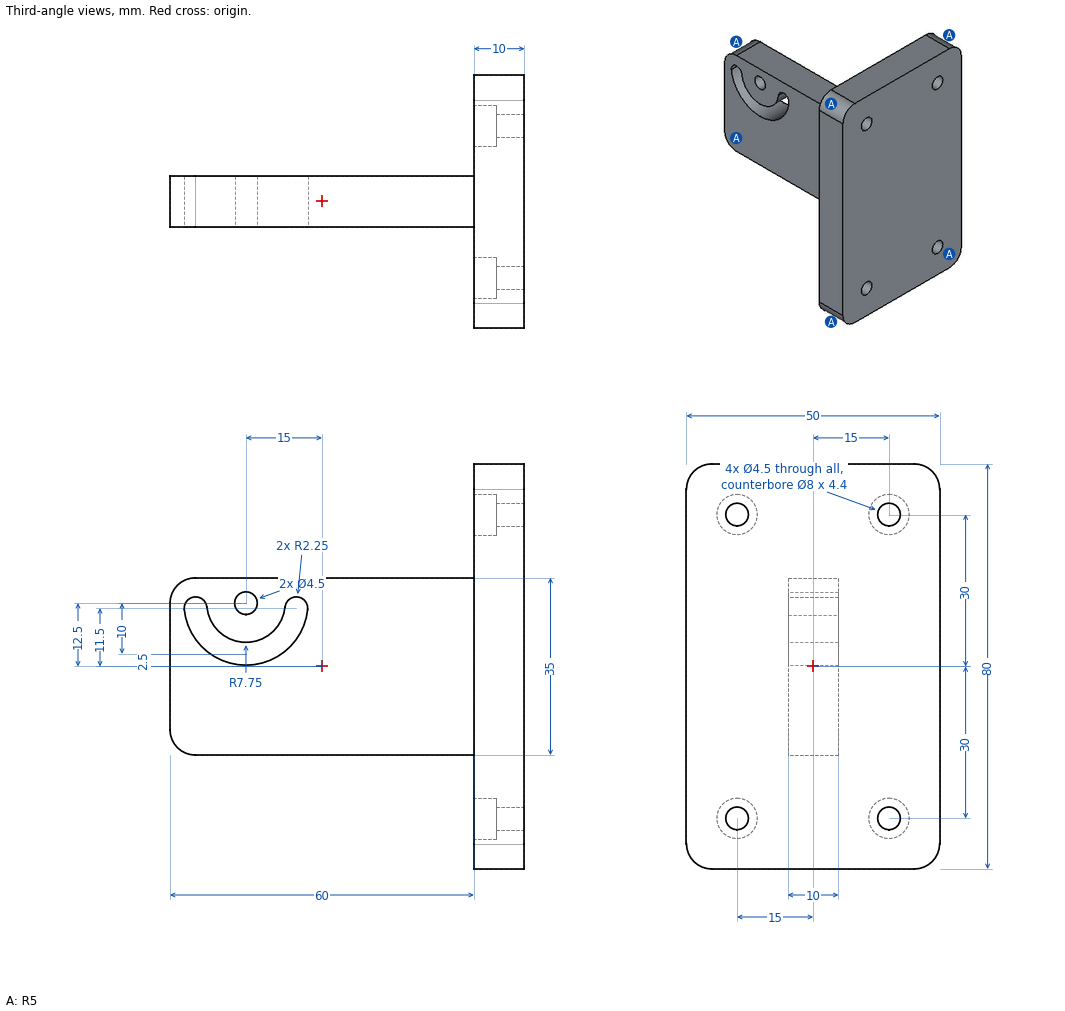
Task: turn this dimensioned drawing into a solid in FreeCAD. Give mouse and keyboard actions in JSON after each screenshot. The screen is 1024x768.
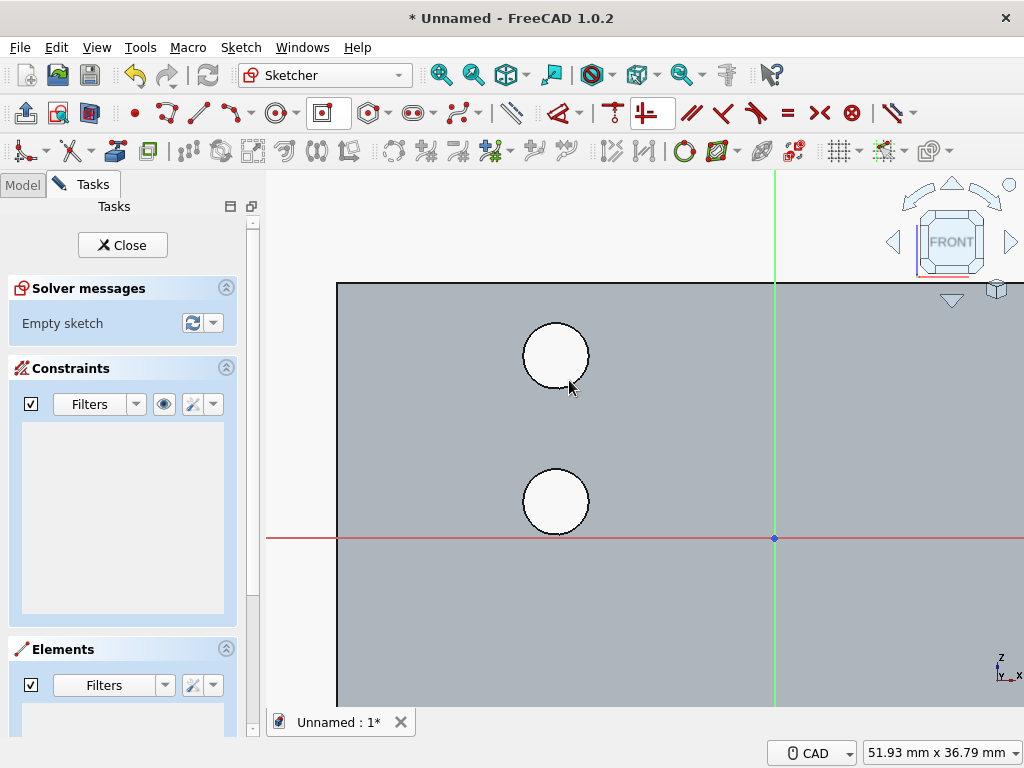
{"action": "left_click", "coordinate": [232, 114]}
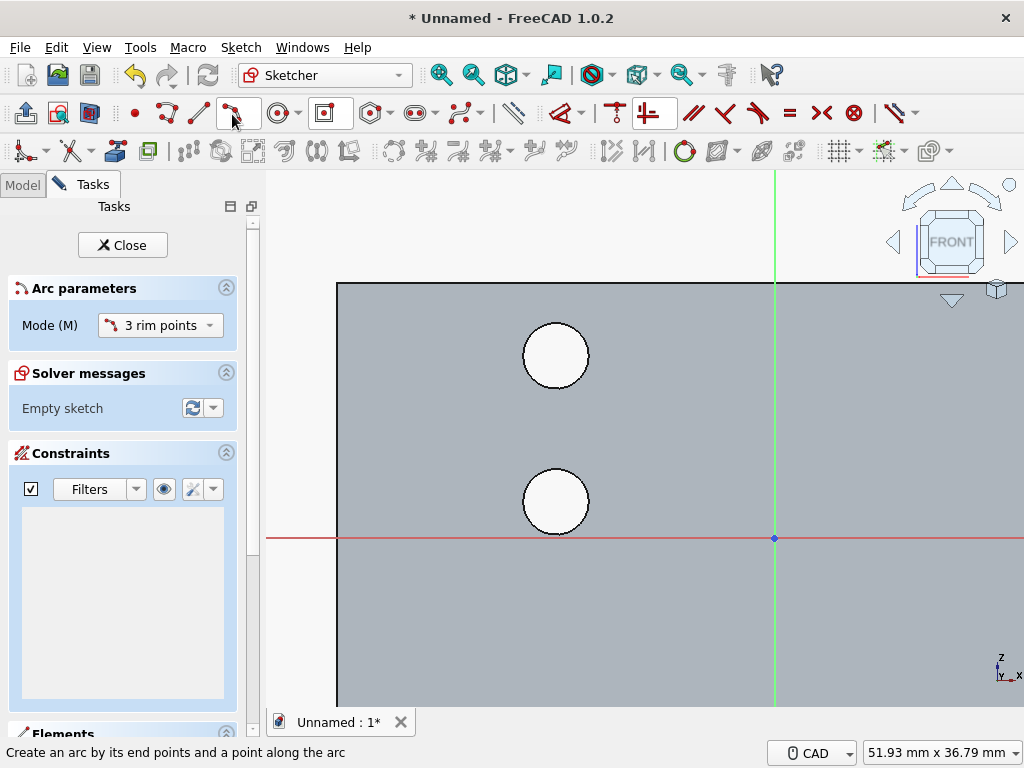
{"action": "left_click", "coordinate": [734, 374]}
{"action": "left_click", "coordinate": [669, 367]}
{"action": "left_click", "coordinate": [704, 338]}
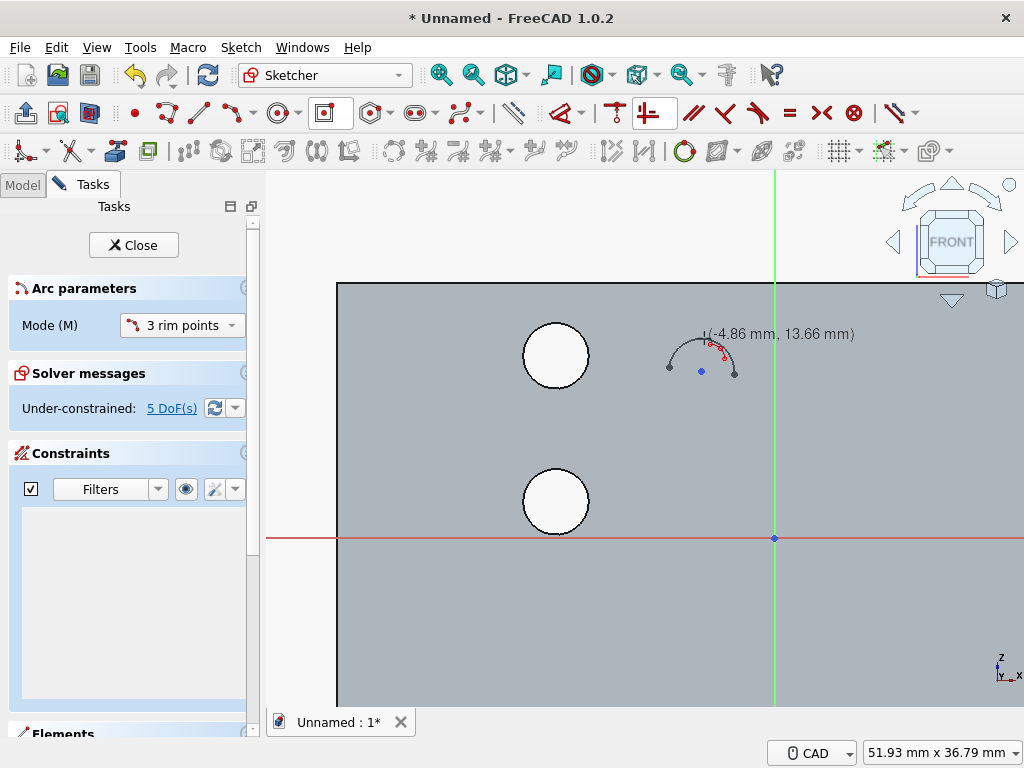
{"action": "left_click", "coordinate": [669, 368]}
{"action": "left_click", "coordinate": [443, 367]}
{"action": "left_click", "coordinate": [556, 469]}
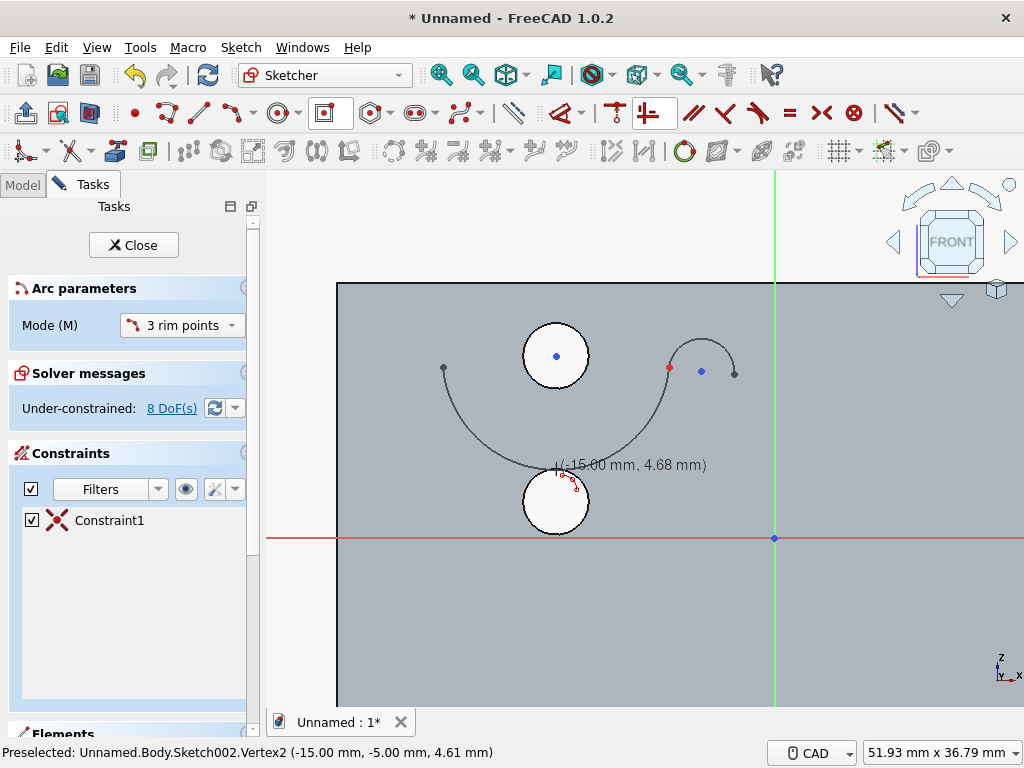
{"action": "left_click", "coordinate": [443, 368]}
{"action": "left_click", "coordinate": [378, 374]}
{"action": "left_click", "coordinate": [407, 338]}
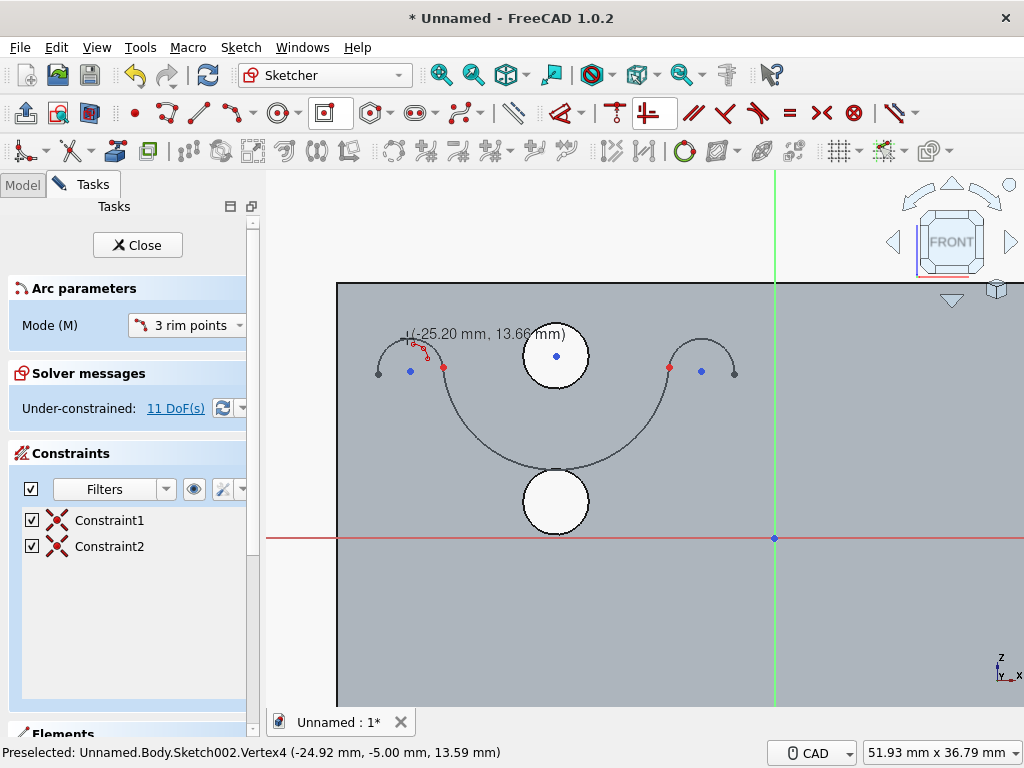
{"action": "left_click", "coordinate": [378, 375]}
{"action": "left_click", "coordinate": [734, 375]}
{"action": "left_click", "coordinate": [457, 505]}
{"action": "key", "text": "Escape"}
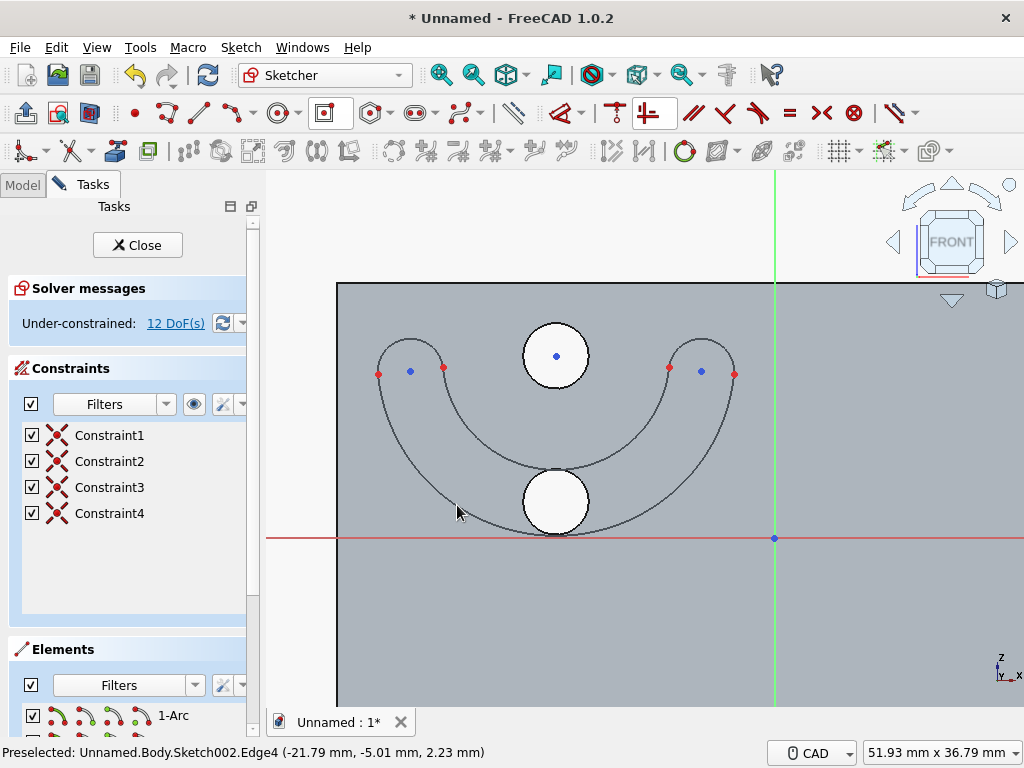
{"action": "left_click", "coordinate": [723, 347]}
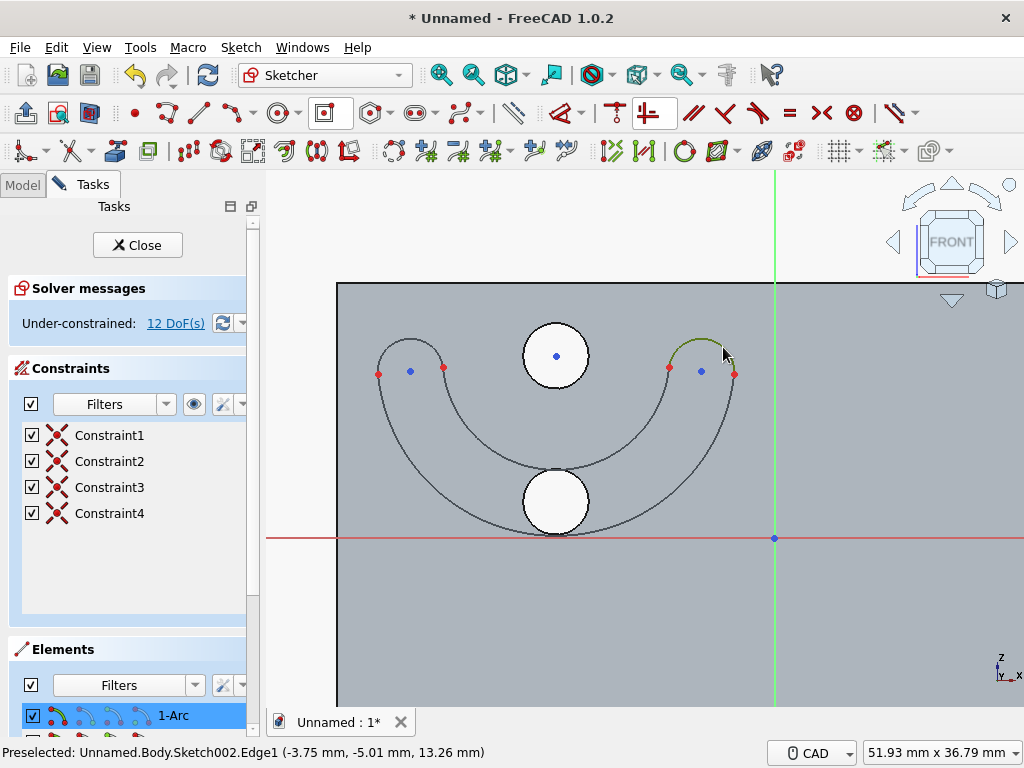
{"action": "left_click", "coordinate": [493, 451]}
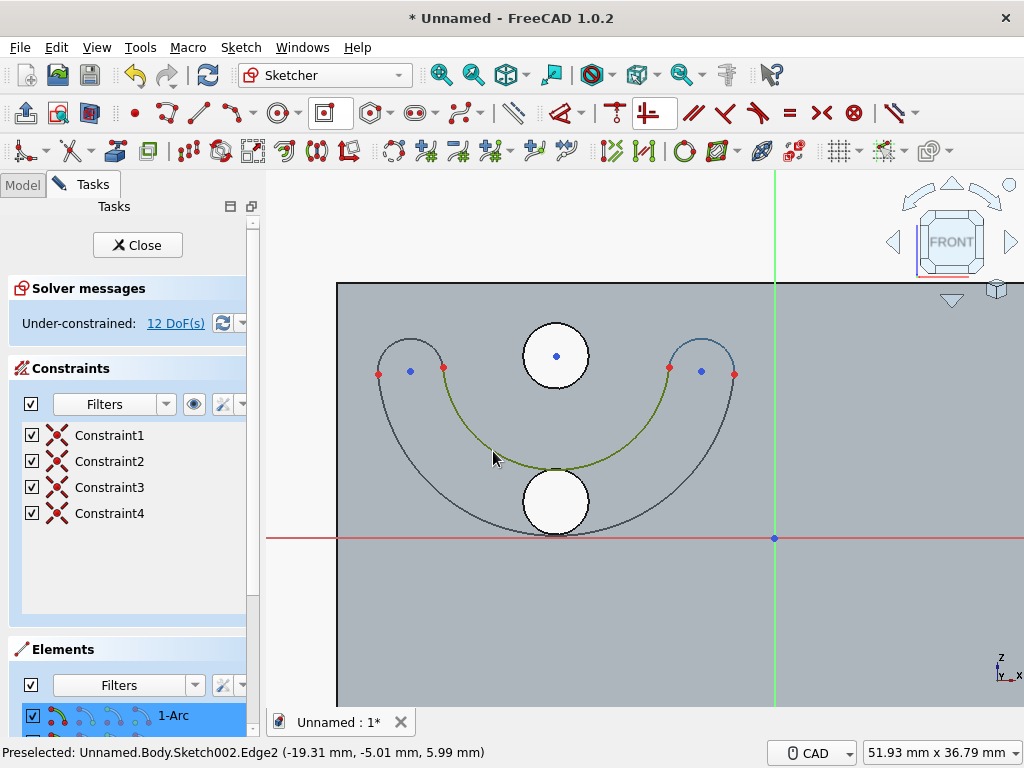
{"action": "left_click", "coordinate": [758, 114]}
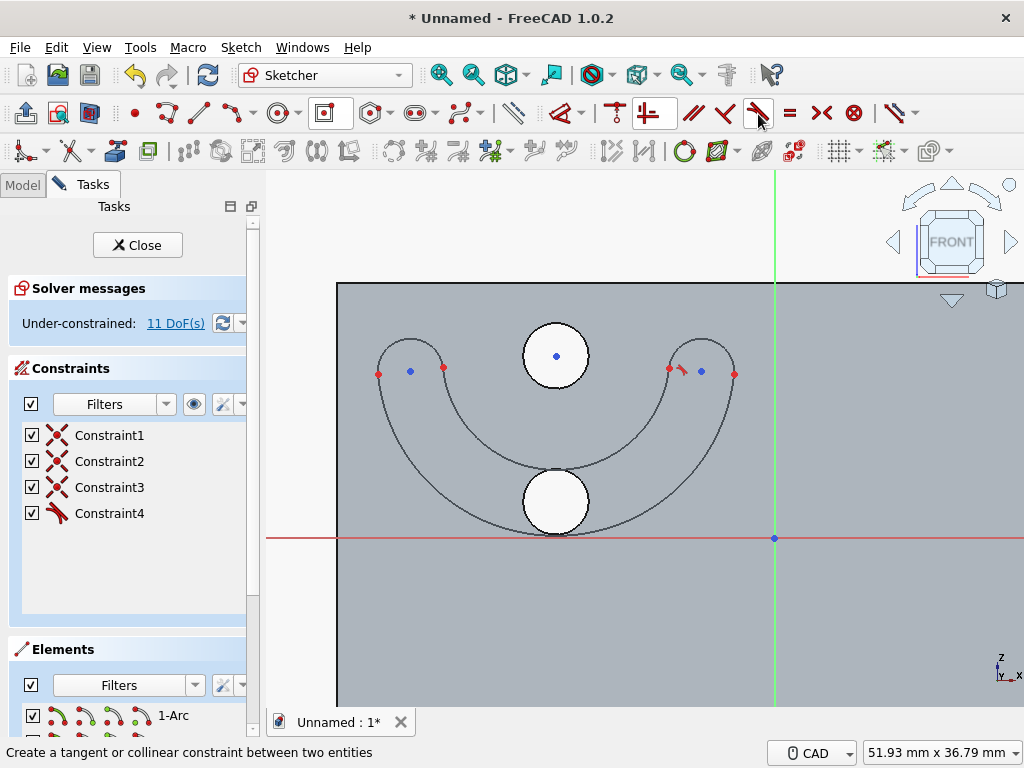
{"action": "left_click", "coordinate": [723, 347]}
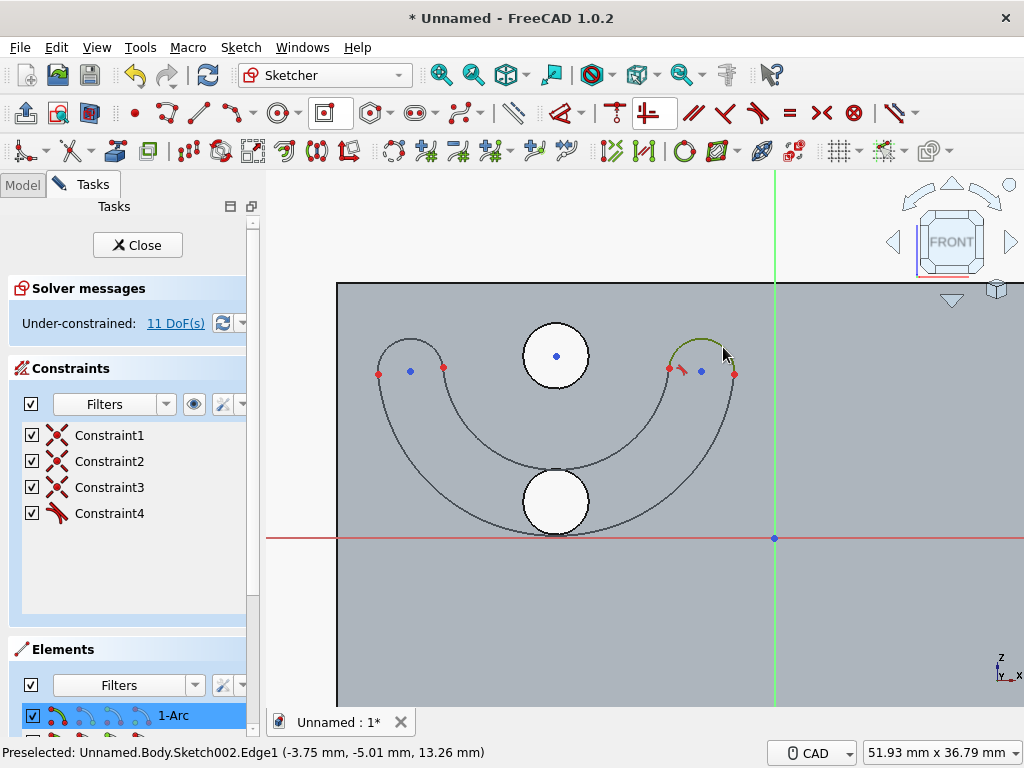
{"action": "left_click", "coordinate": [457, 506]}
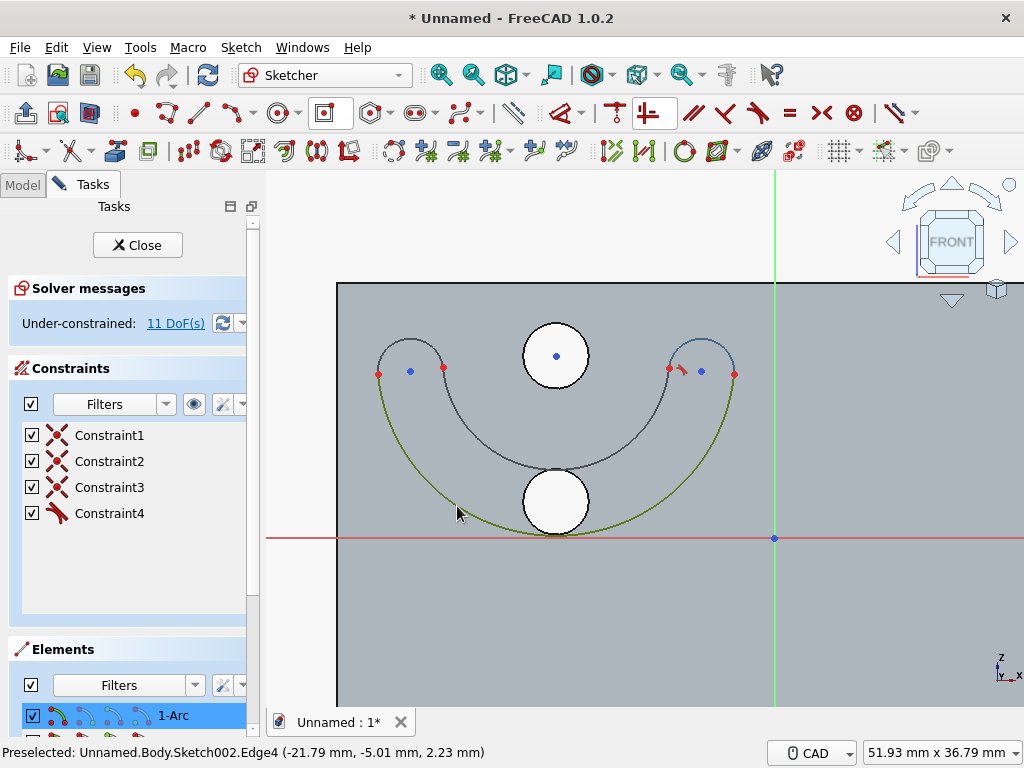
{"action": "left_click", "coordinate": [758, 114]}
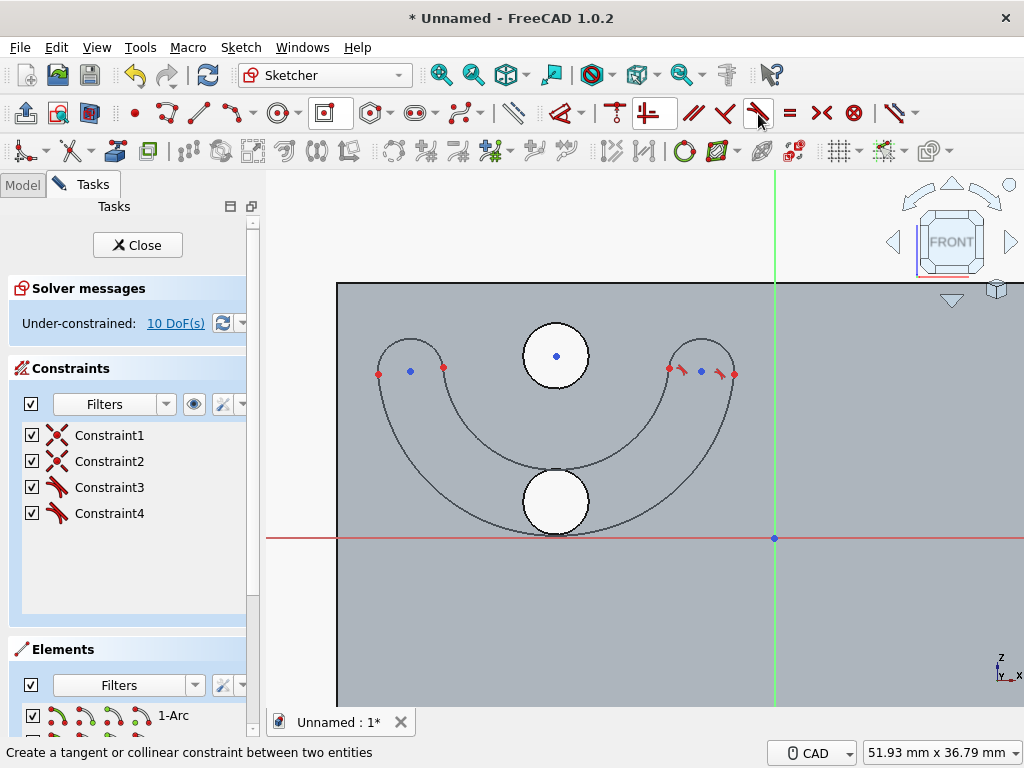
{"action": "left_click", "coordinate": [493, 451]}